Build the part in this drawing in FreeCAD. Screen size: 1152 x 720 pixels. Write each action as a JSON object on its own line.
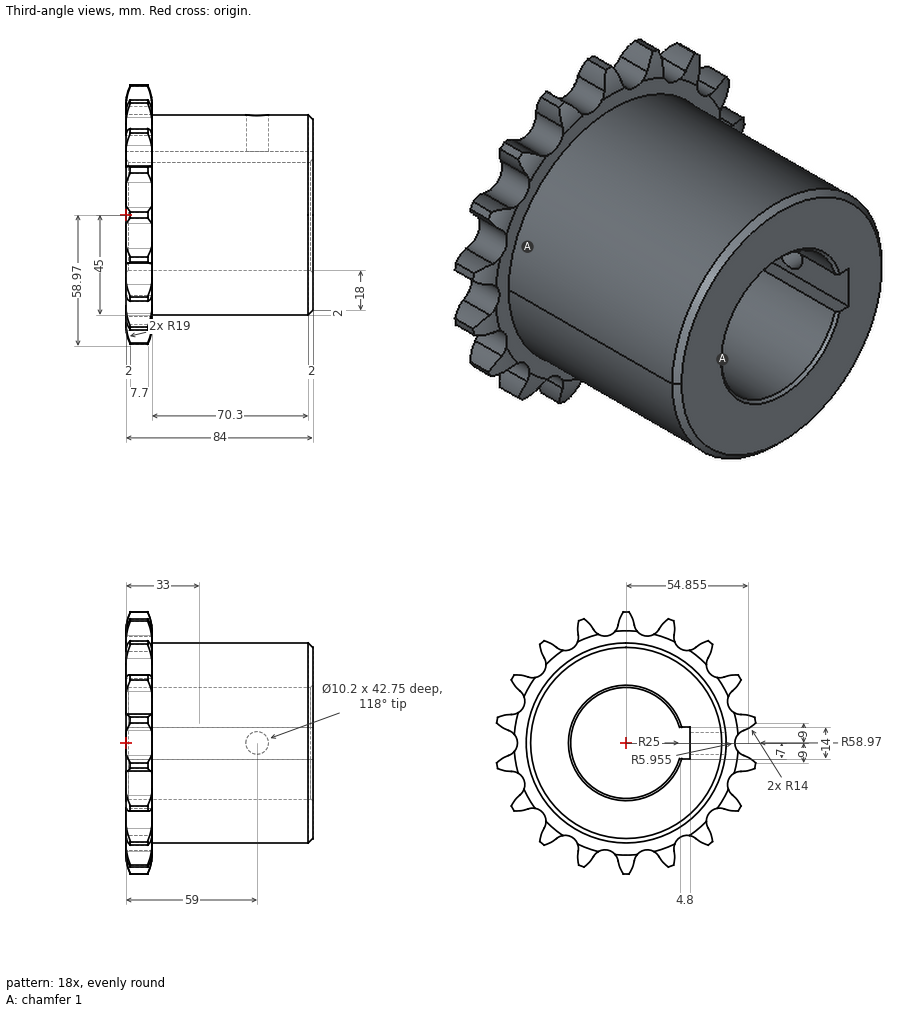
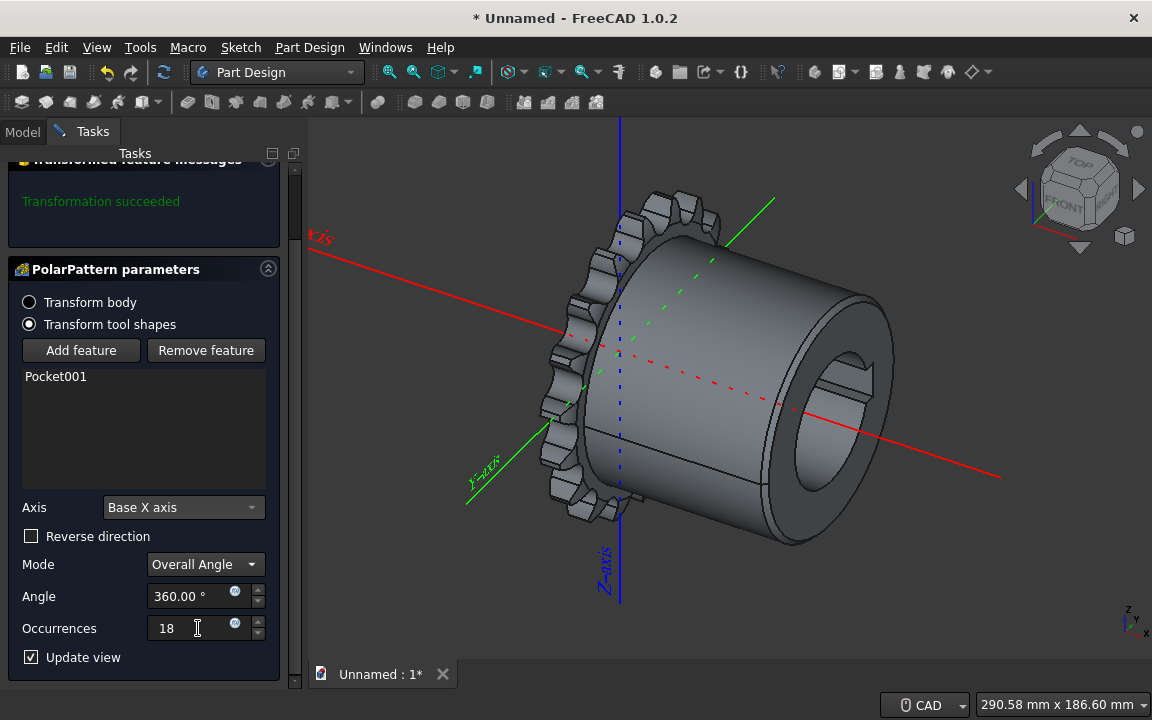
{"action": "scroll", "coordinate": [295, 426], "scroll_direction": "up", "scroll_amount": 3}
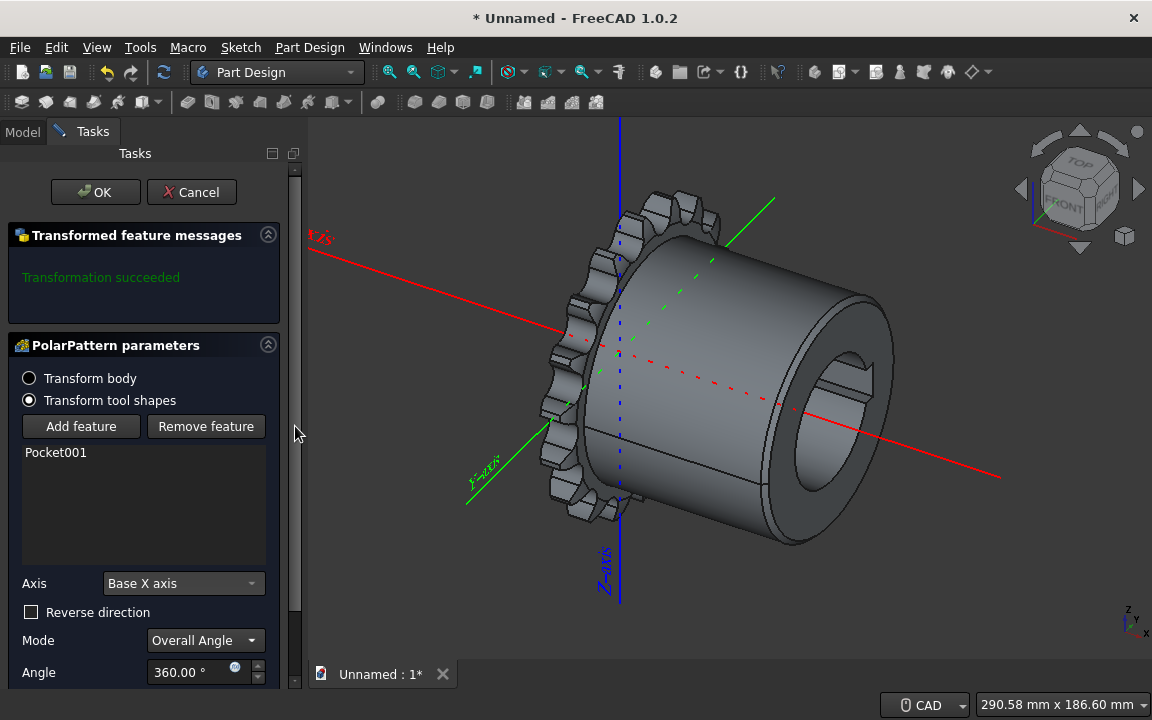
{"action": "left_click", "coordinate": [96, 192]}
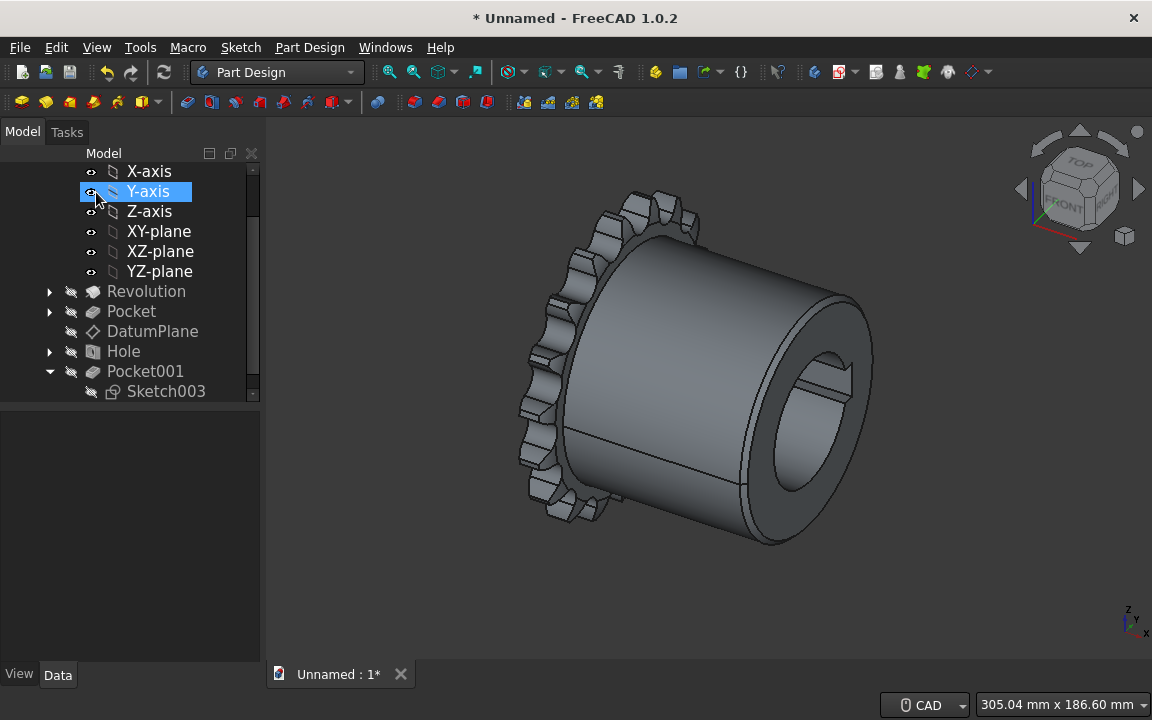
{"action": "left_click", "coordinate": [805, 485]}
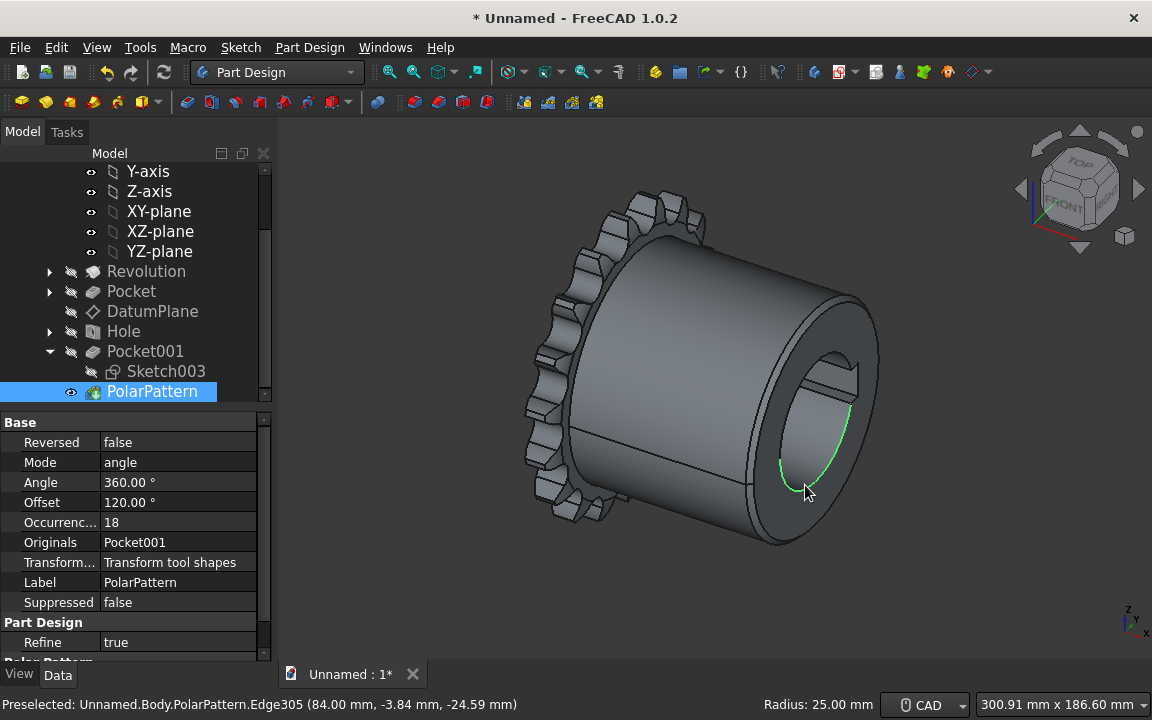
{"action": "key", "text": "0"}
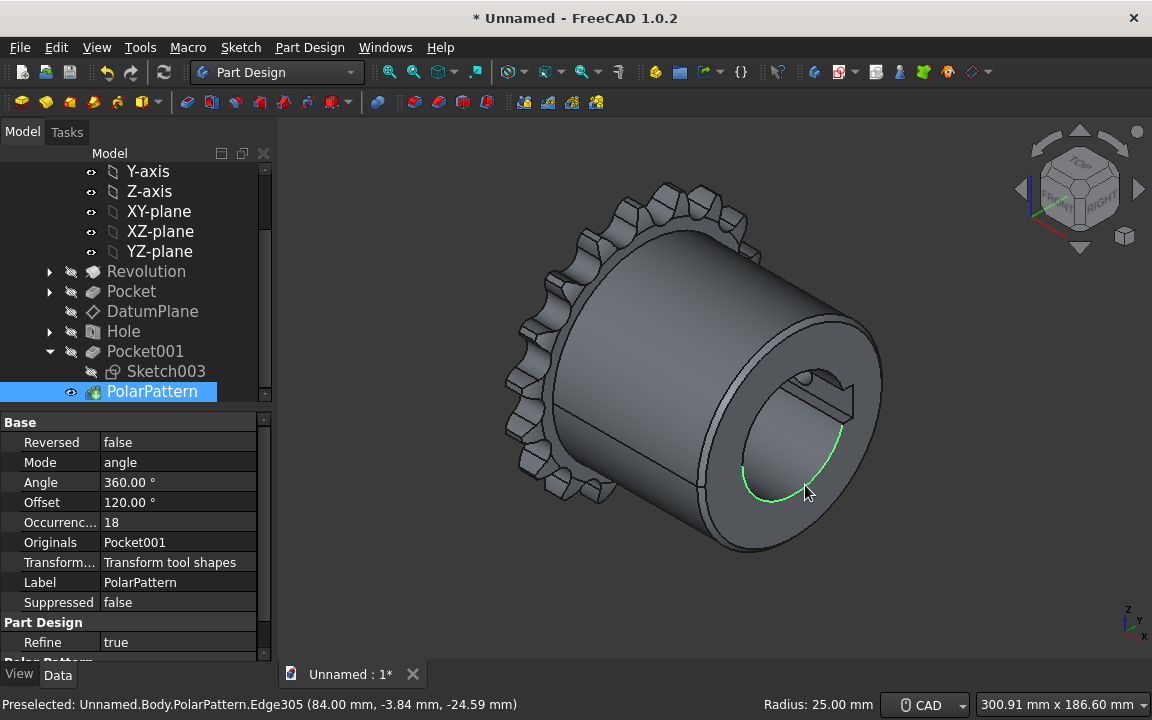
{"action": "key", "text": "2"}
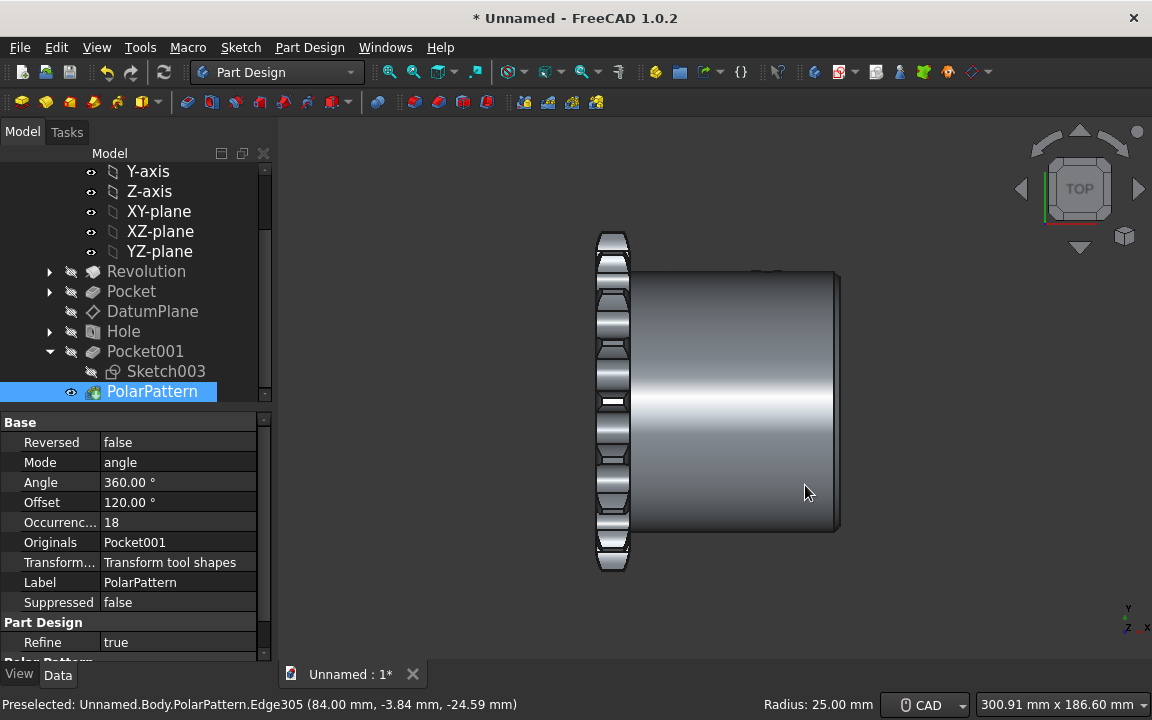
{"action": "key", "text": "1"}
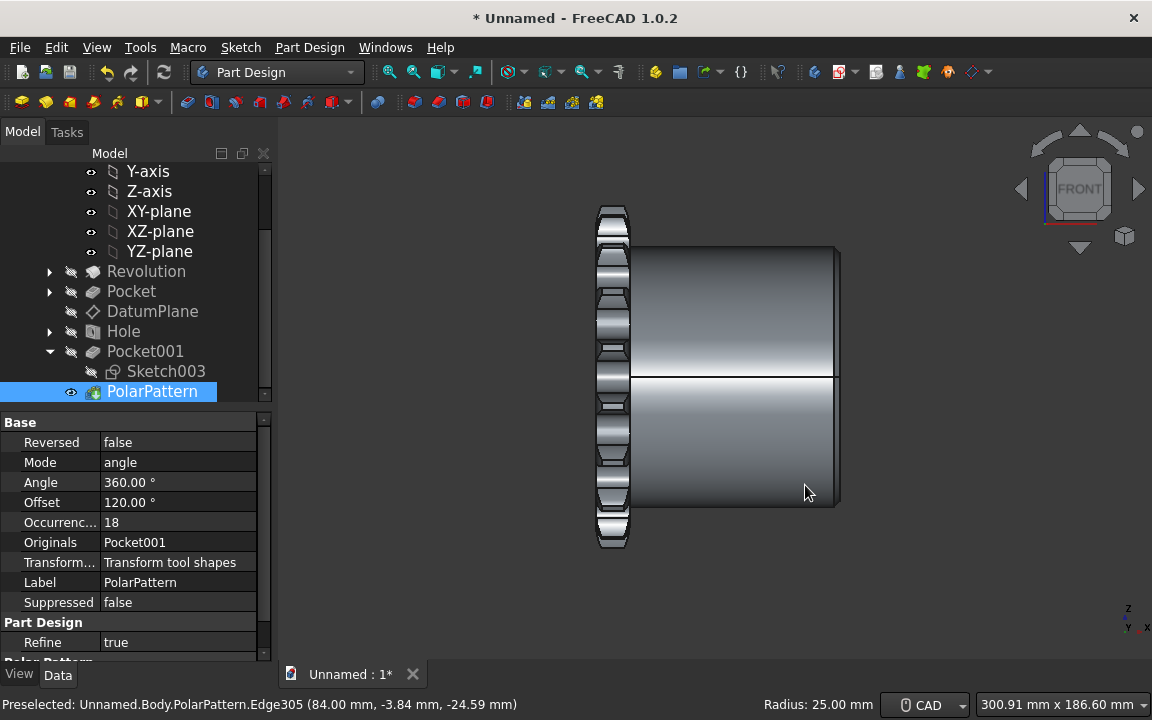
{"action": "key", "text": "3"}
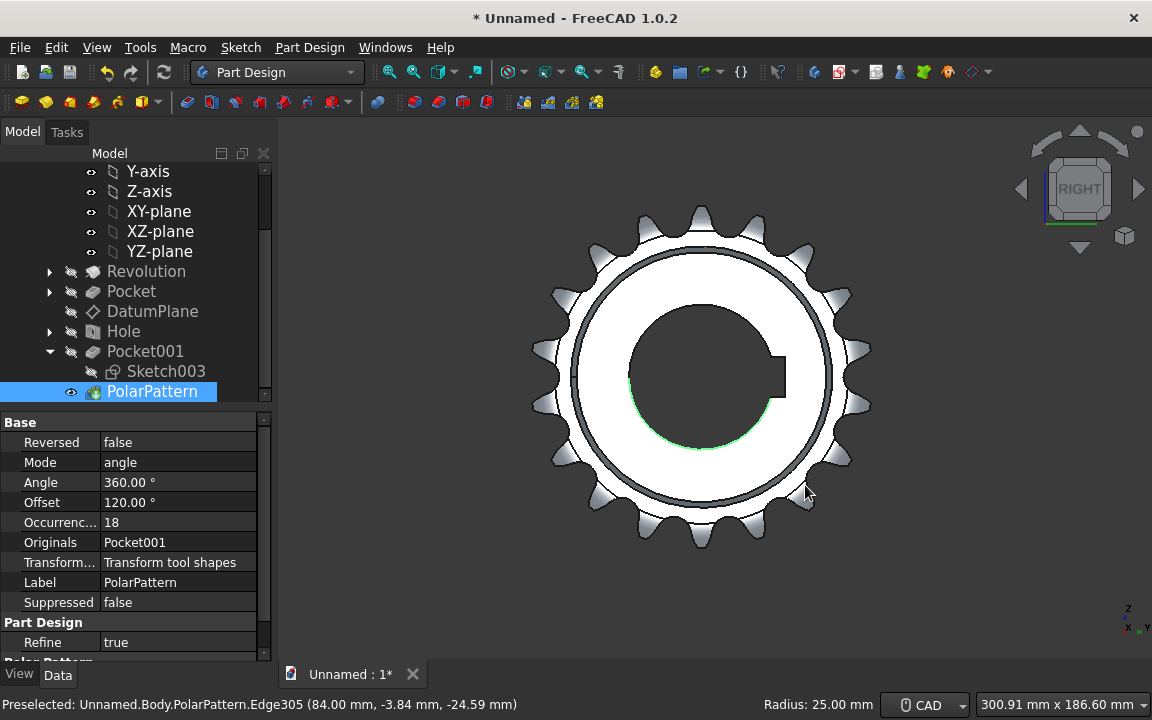
{"action": "key", "text": "5"}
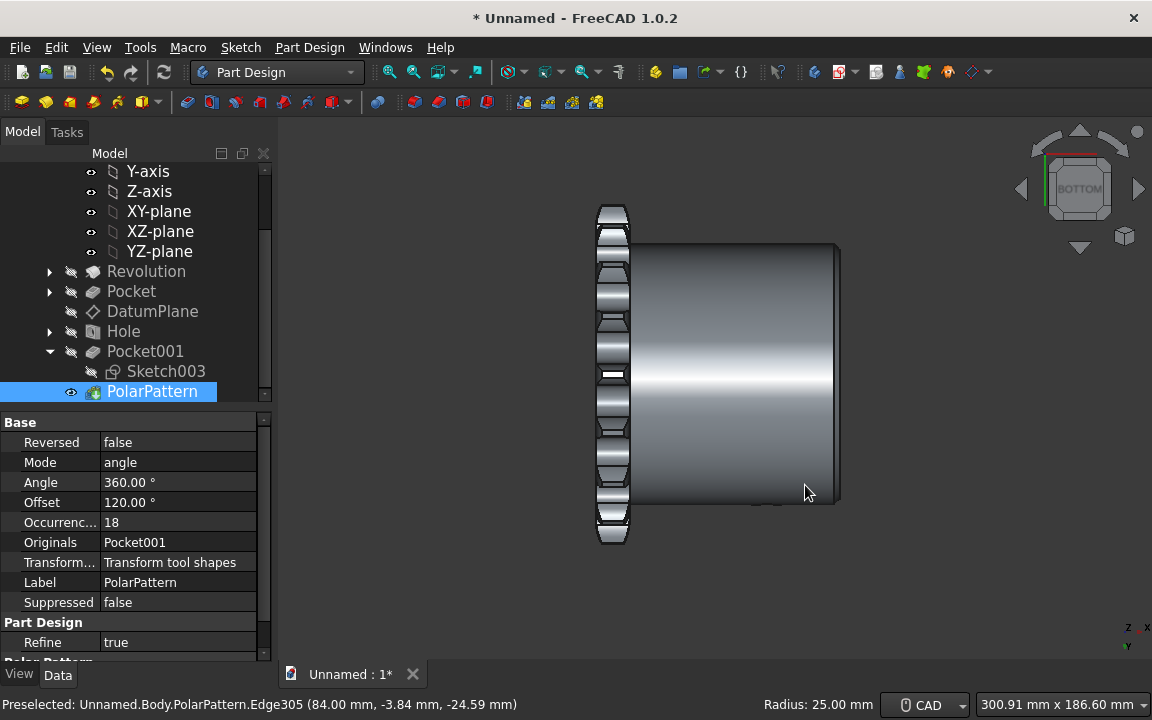
{"action": "key", "text": "4"}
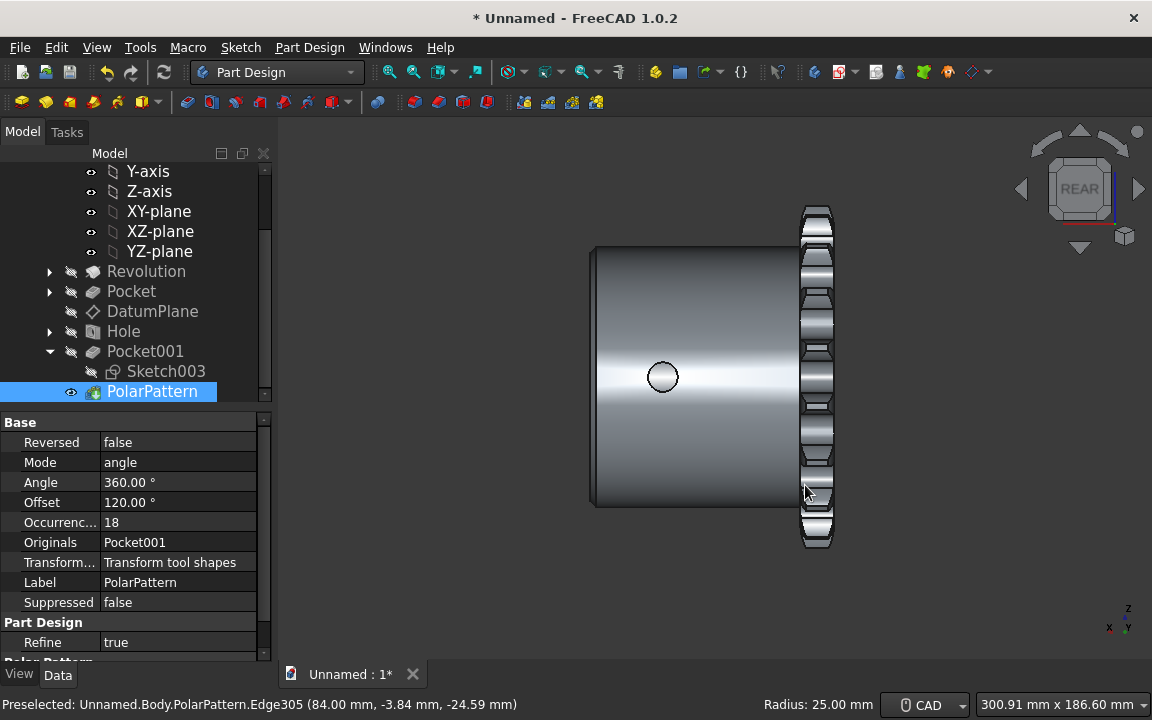
{"action": "key", "text": "6"}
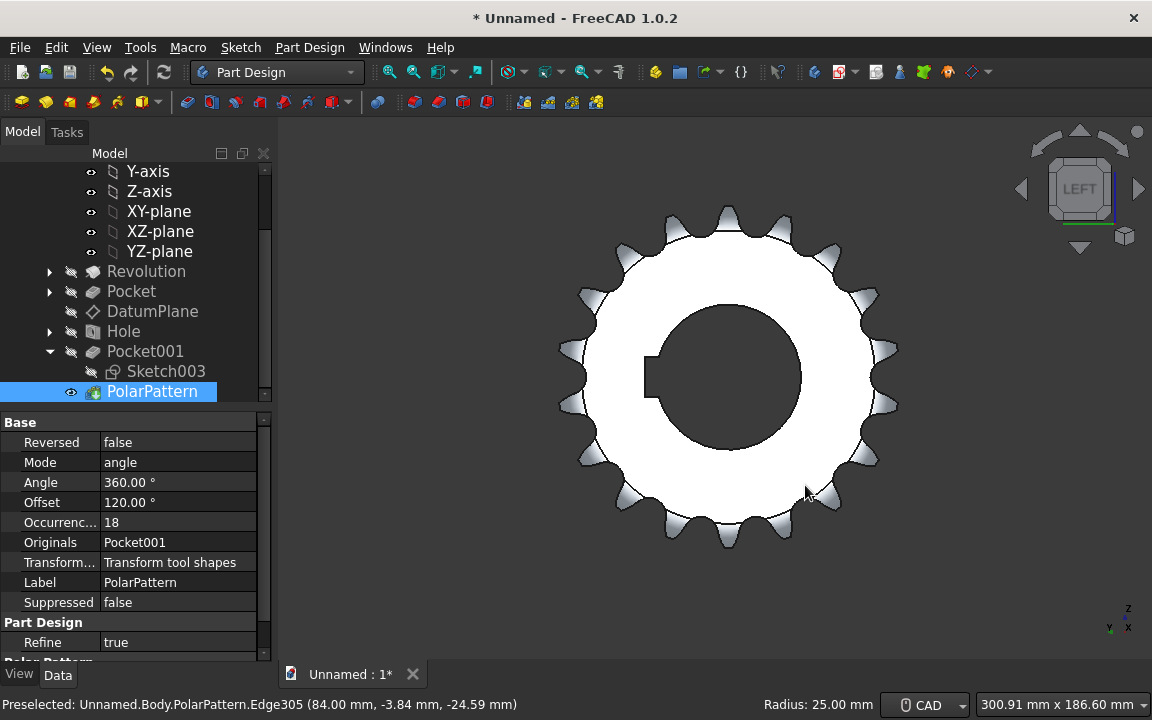
{"action": "left_click", "coordinate": [739, 448], "text": "ctrl"}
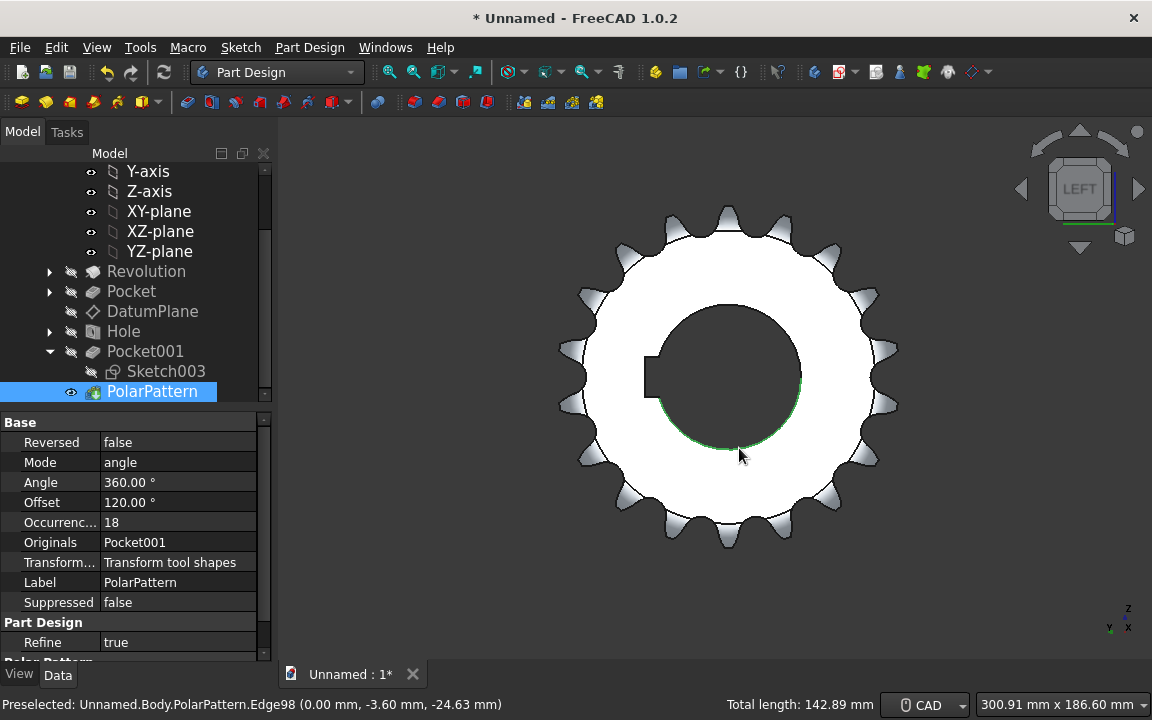
{"action": "left_click", "coordinate": [440, 102]}